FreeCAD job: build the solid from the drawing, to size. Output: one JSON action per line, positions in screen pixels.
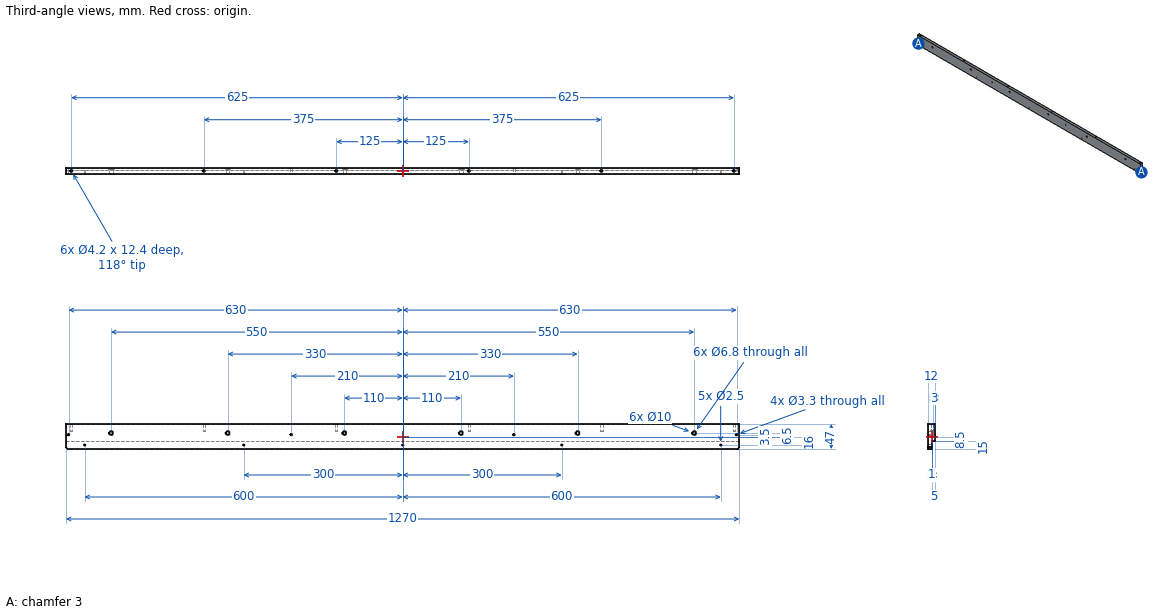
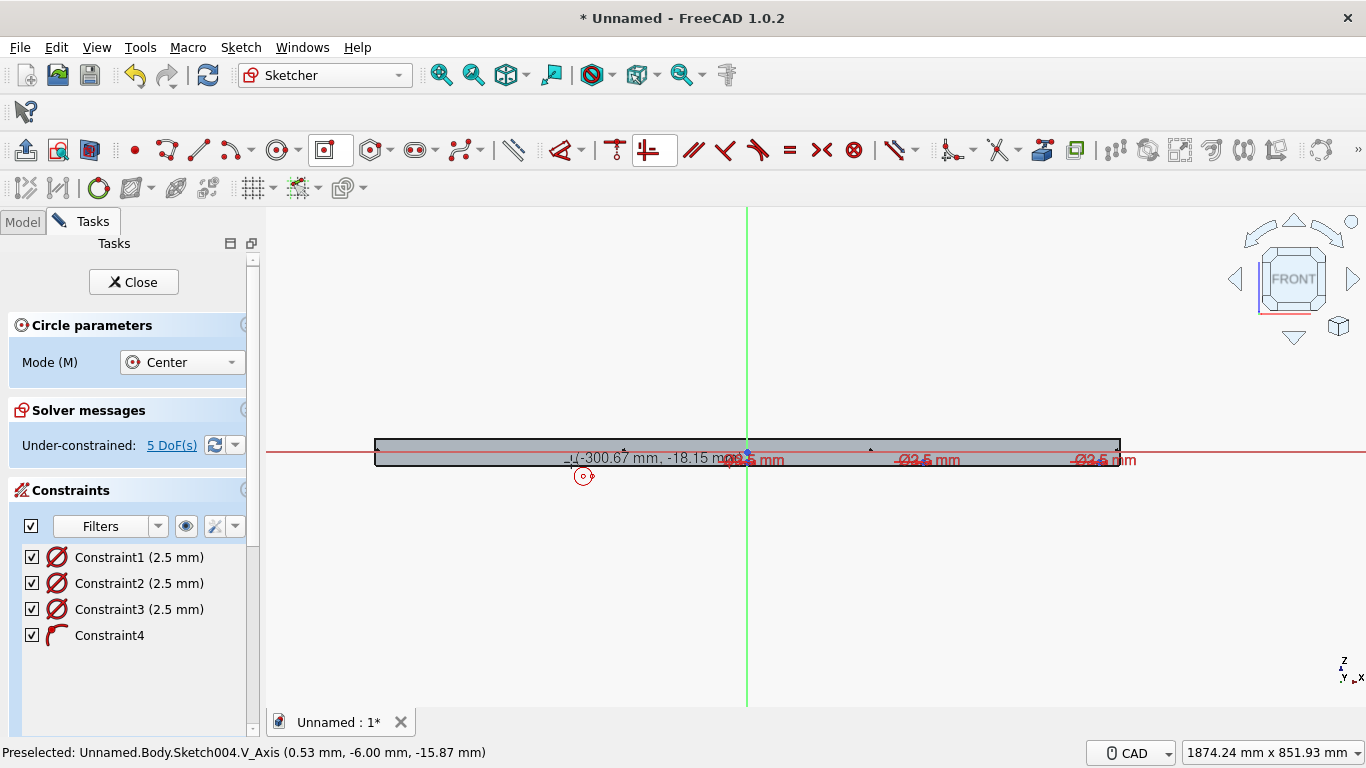
{"action": "scroll", "coordinate": [571, 462], "scroll_direction": "up", "scroll_amount": 3}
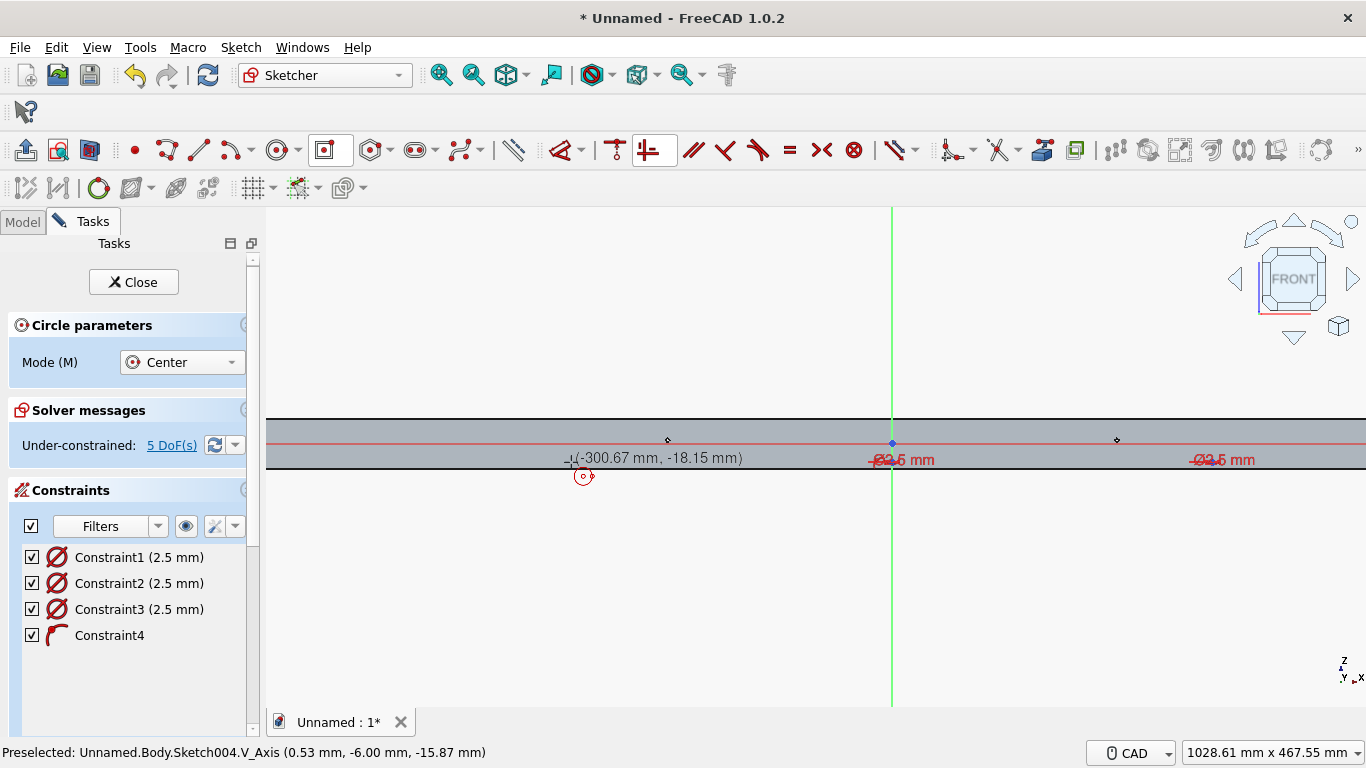
{"action": "left_click", "coordinate": [571, 461]}
{"action": "mouse_move", "coordinate": [572, 460]}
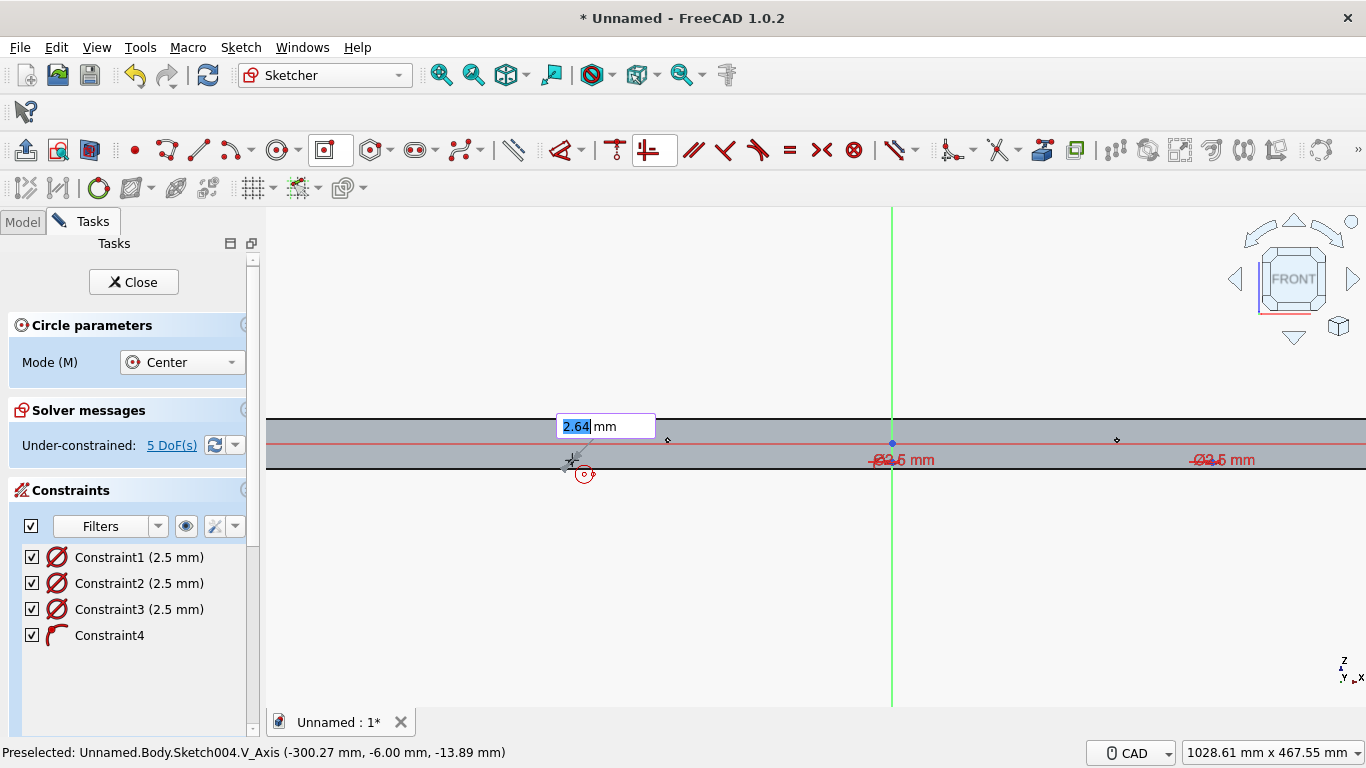
{"action": "type", "text": "2.5"}
{"action": "key", "text": "Return"}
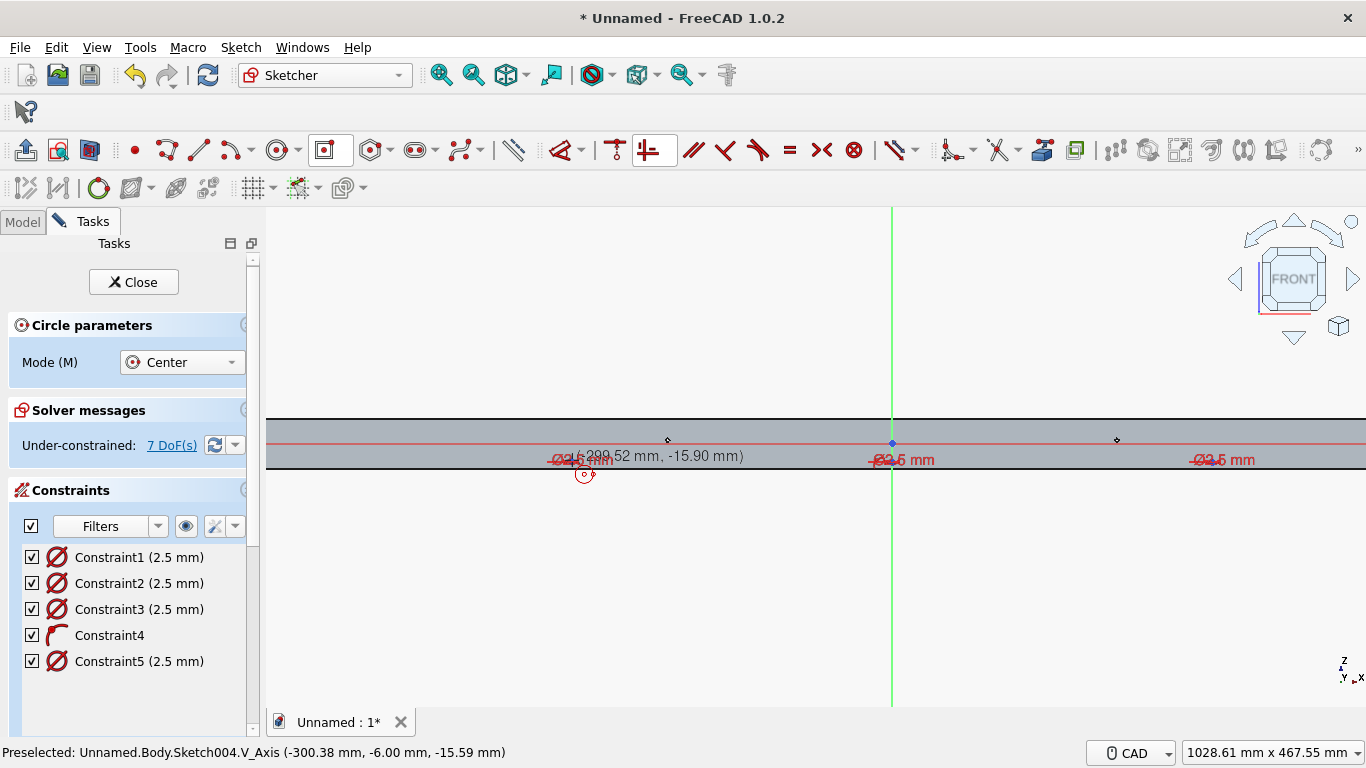
{"action": "scroll", "coordinate": [571, 462], "scroll_direction": "down", "scroll_amount": 3}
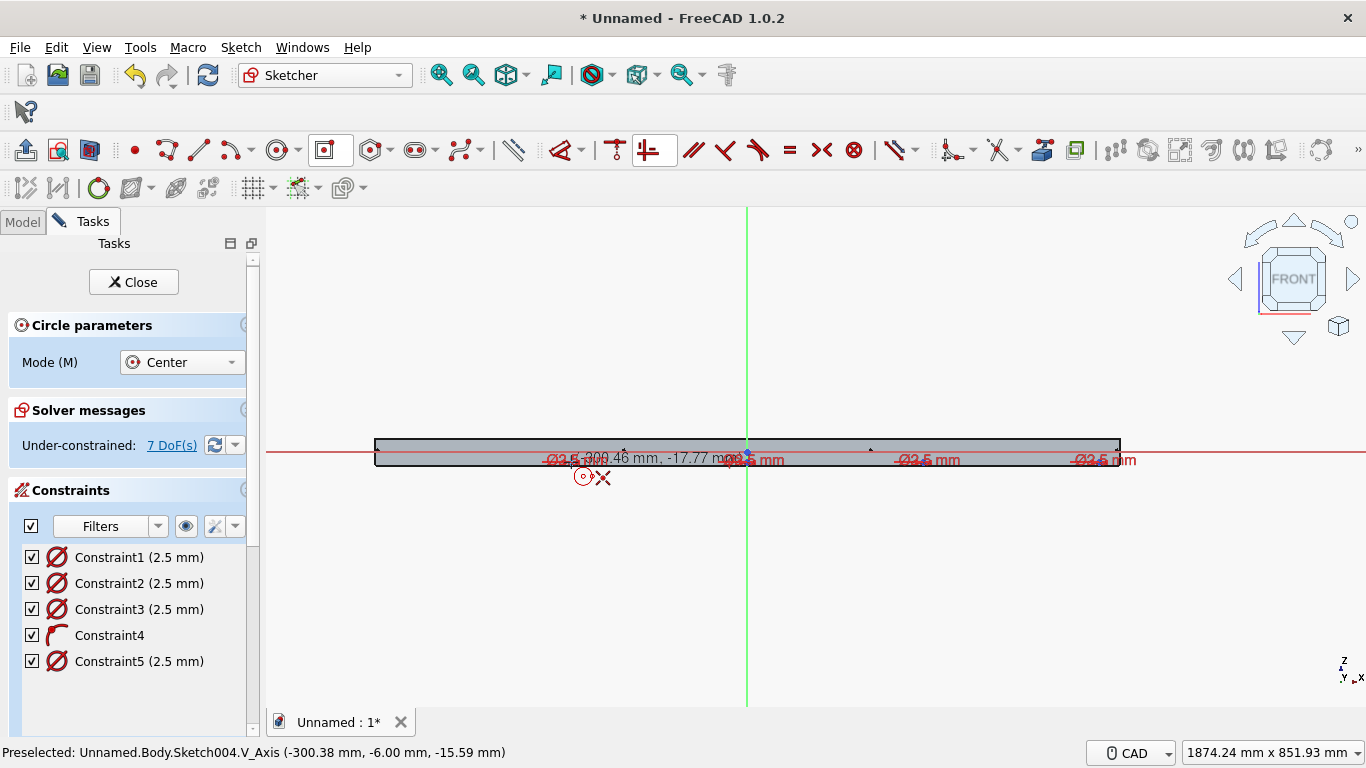
{"action": "scroll", "coordinate": [395, 462], "scroll_direction": "up", "scroll_amount": 18}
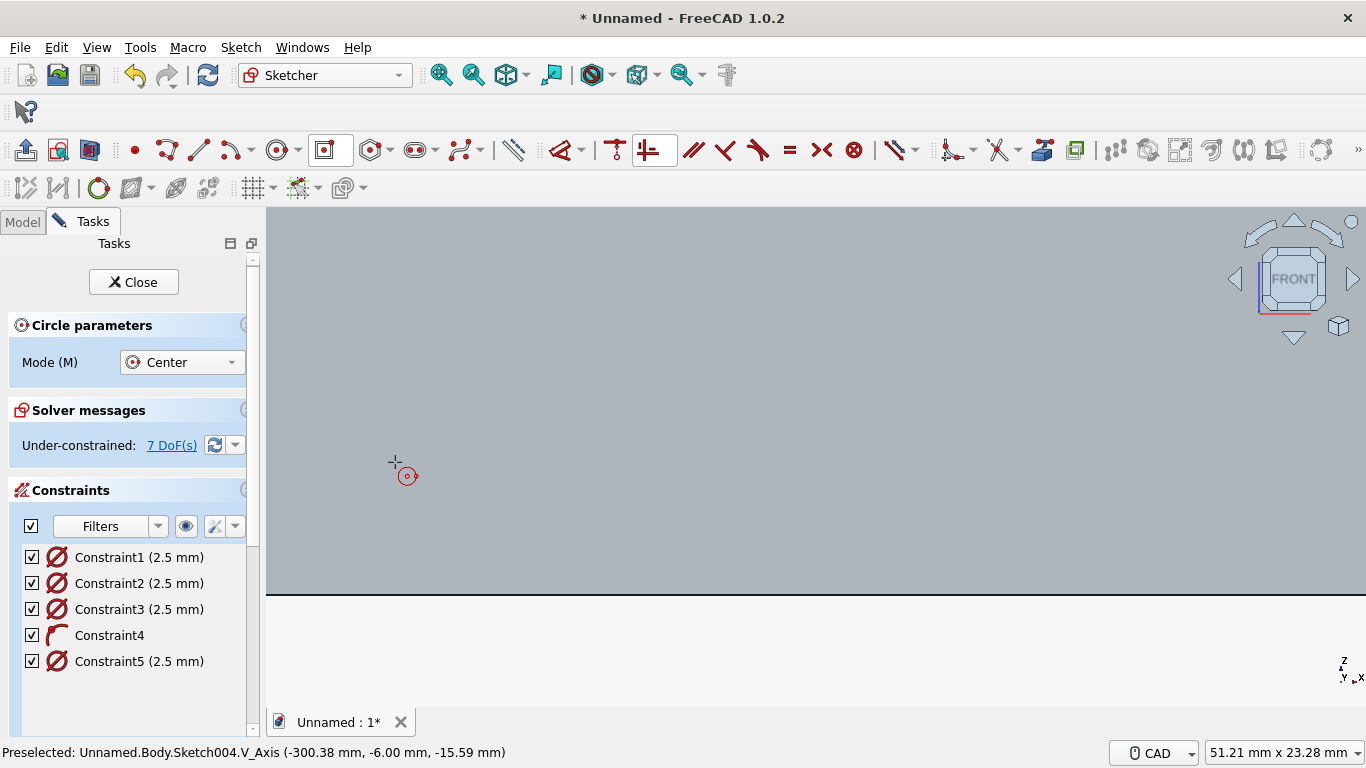
{"action": "scroll", "coordinate": [395, 462], "scroll_direction": "down", "scroll_amount": 18}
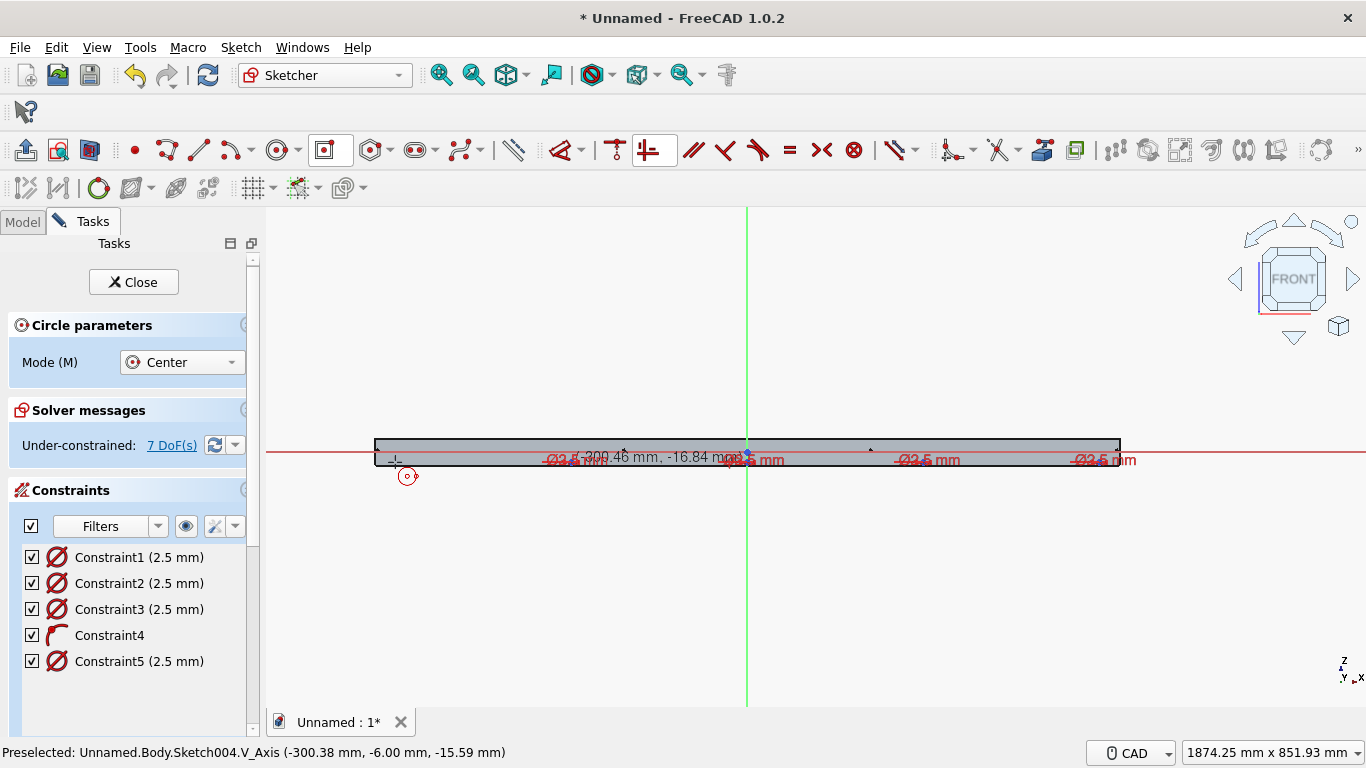
{"action": "scroll", "coordinate": [395, 462], "scroll_direction": "up", "scroll_amount": 3}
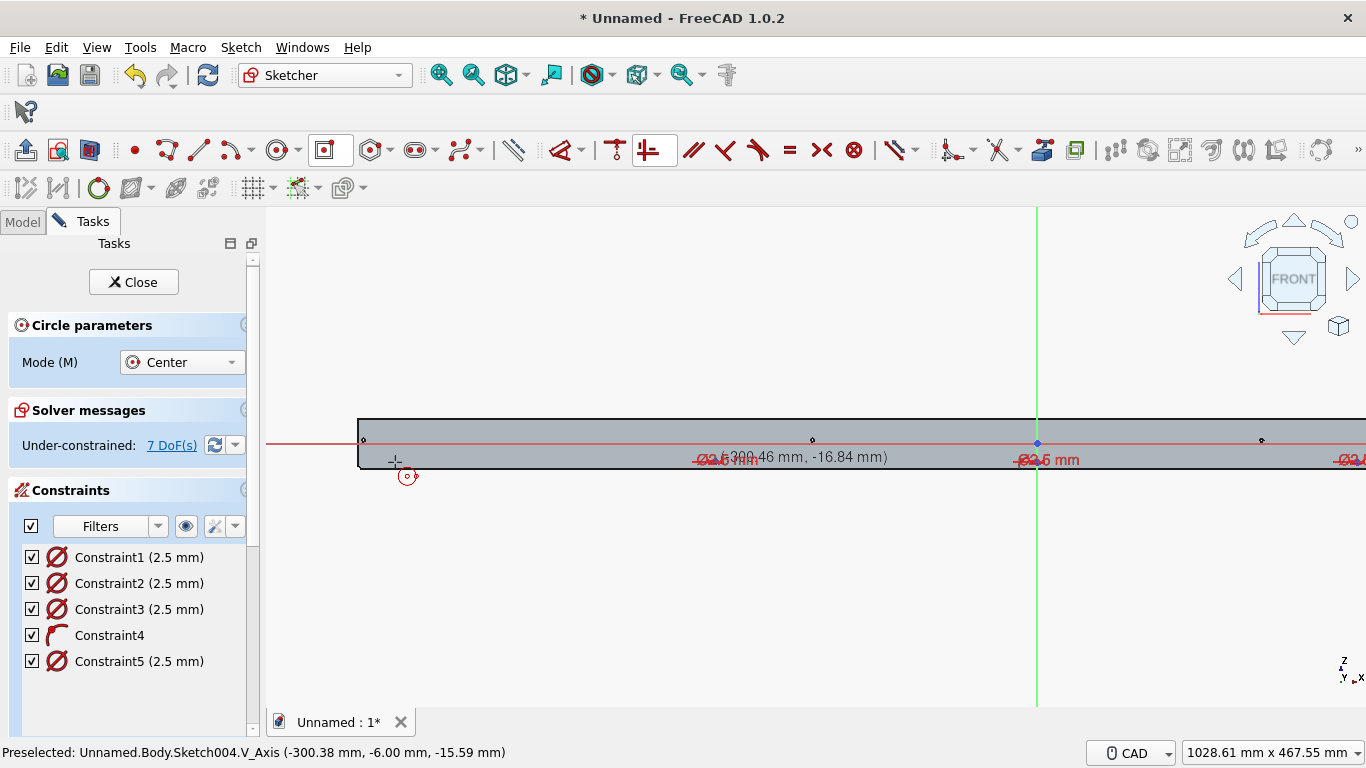
{"action": "left_click", "coordinate": [395, 461]}
{"action": "mouse_move", "coordinate": [396, 460]}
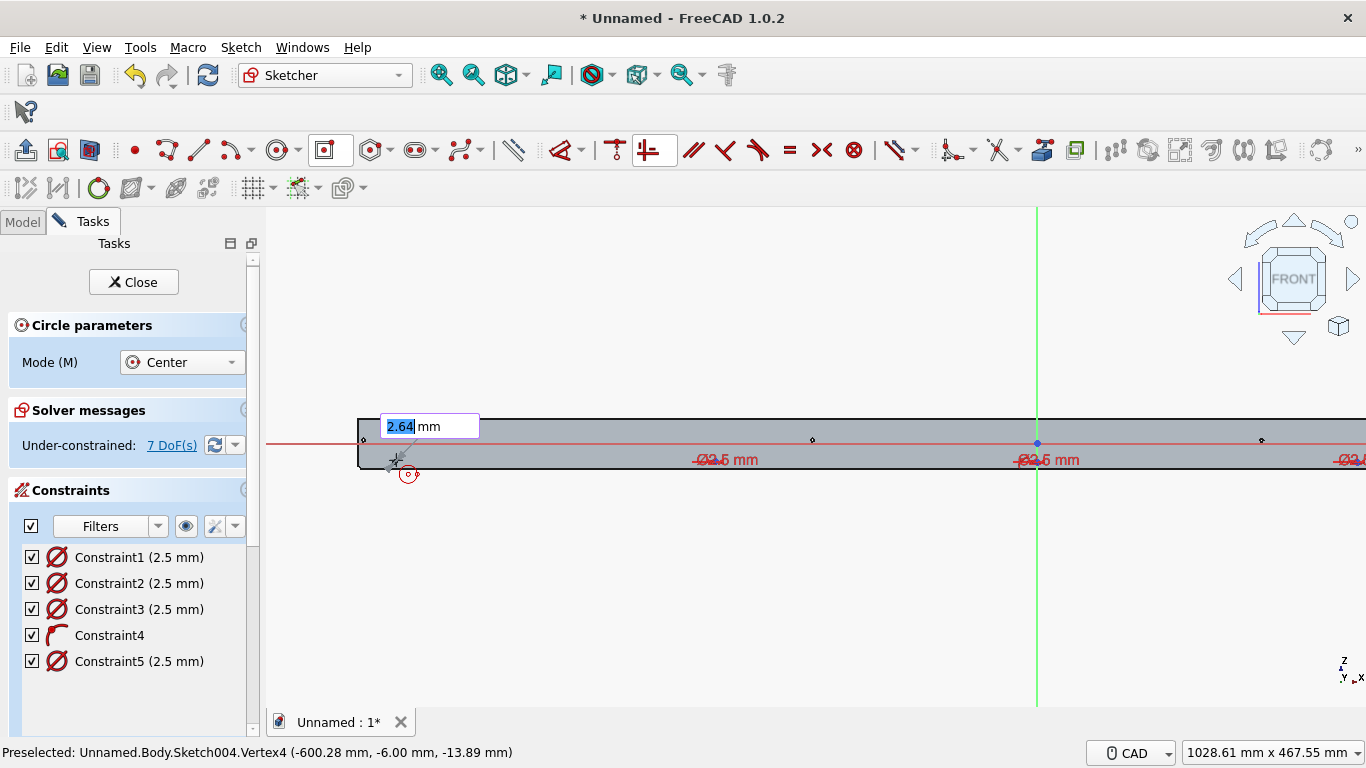
{"action": "type", "text": "2.5"}
{"action": "key", "text": "Return"}
{"action": "key", "text": "Escape"}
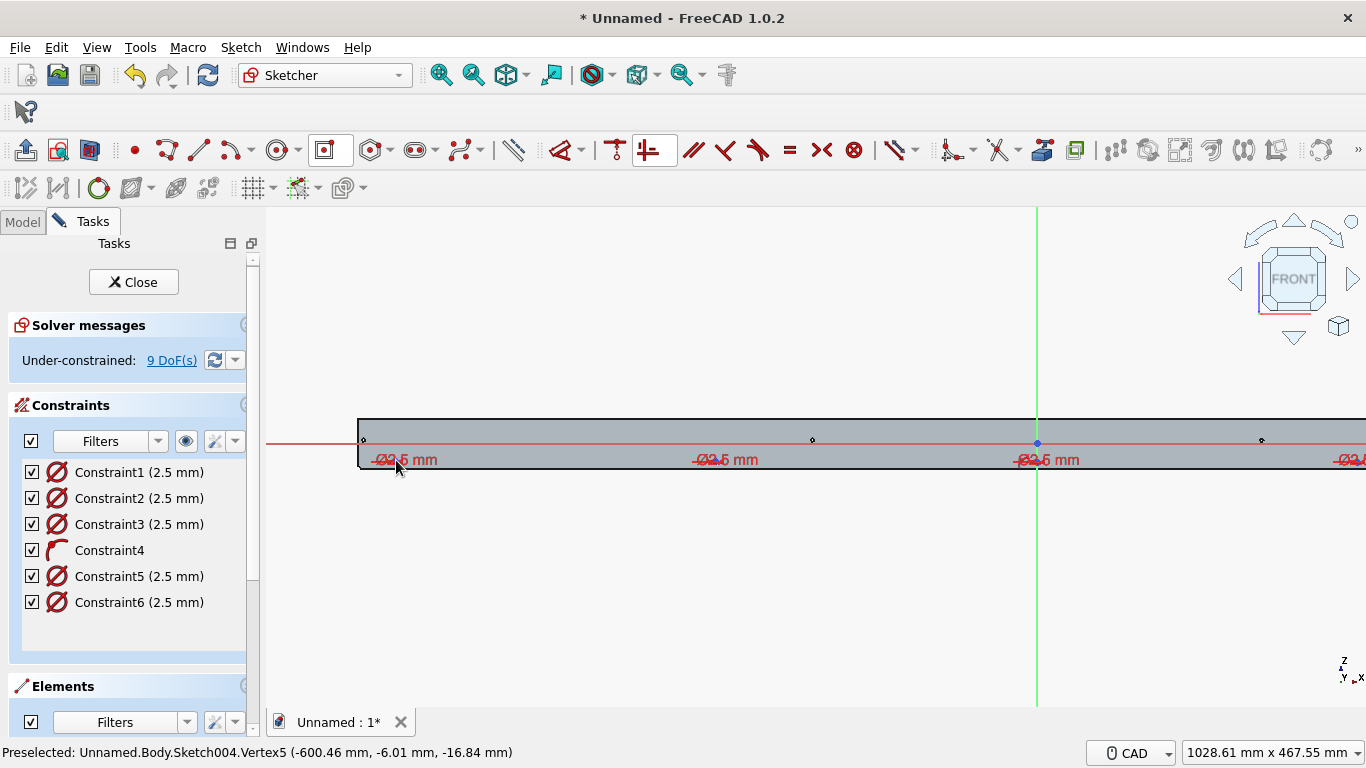
{"action": "scroll", "coordinate": [395, 462], "scroll_direction": "down", "scroll_amount": 3}